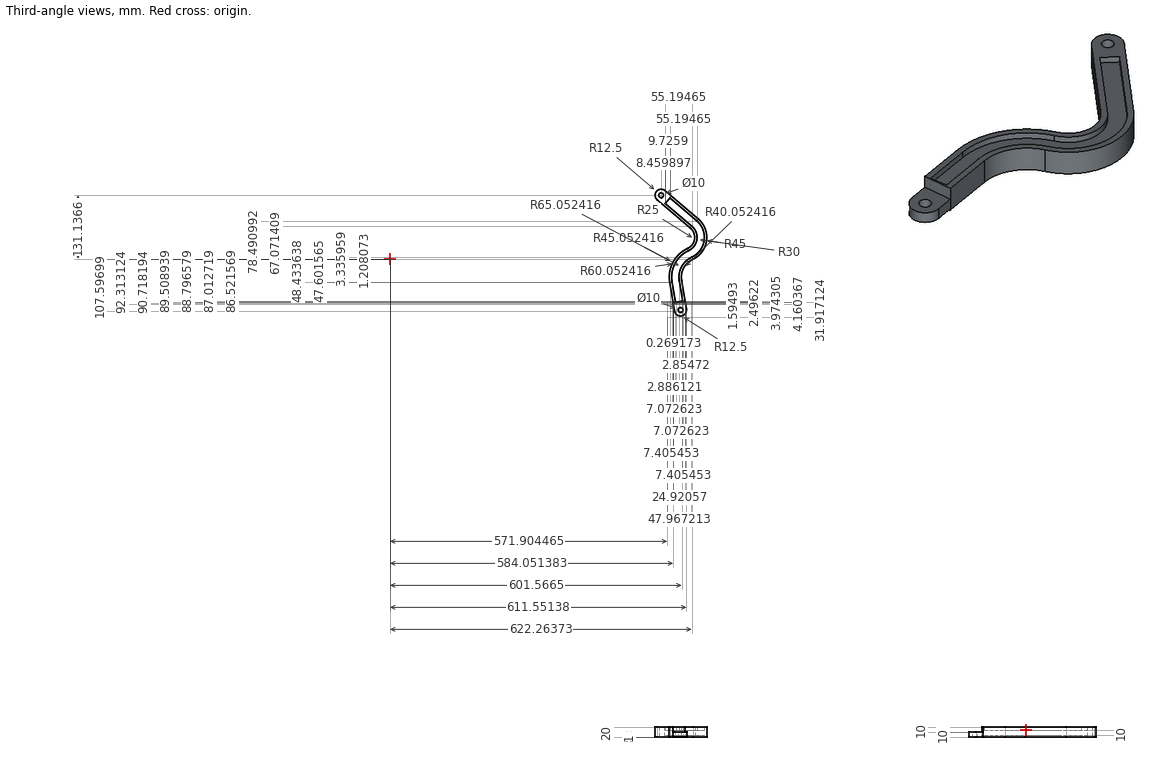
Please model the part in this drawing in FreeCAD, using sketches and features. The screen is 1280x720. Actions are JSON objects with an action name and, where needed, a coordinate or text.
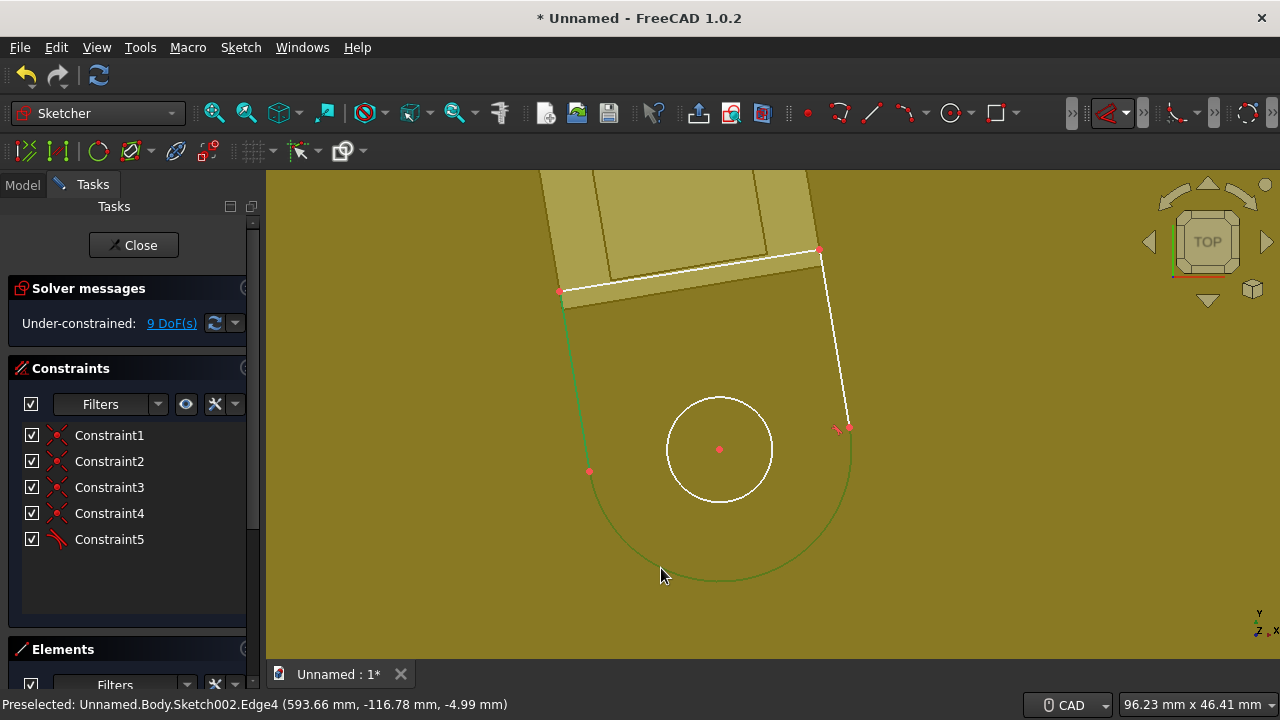
{"action": "key", "text": "t"}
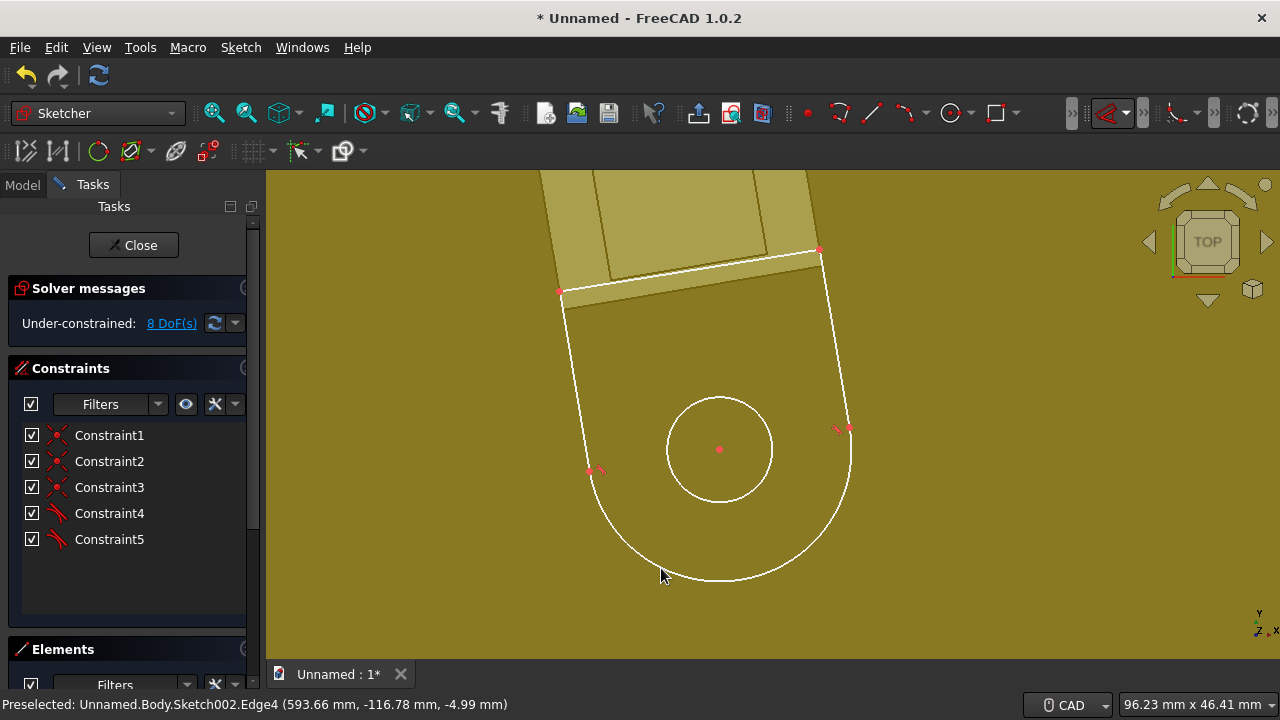
{"action": "left_click", "coordinate": [661, 568]}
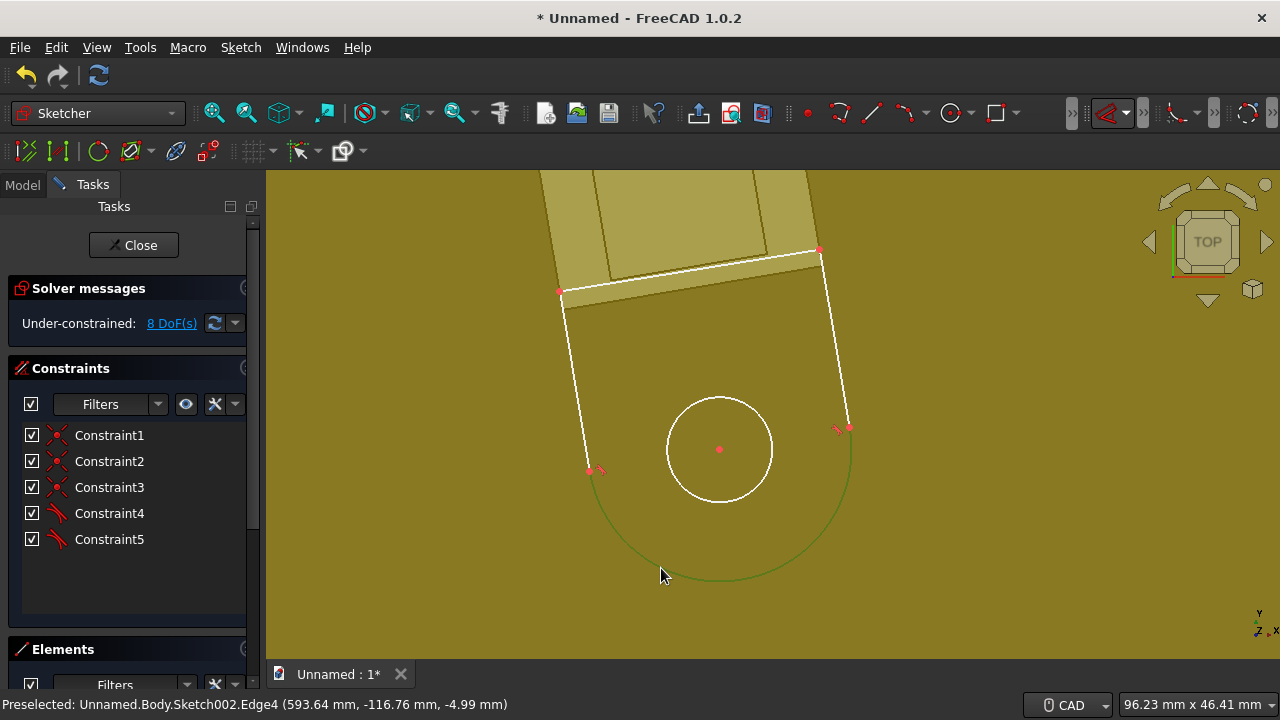
{"action": "left_click", "coordinate": [1128, 114]}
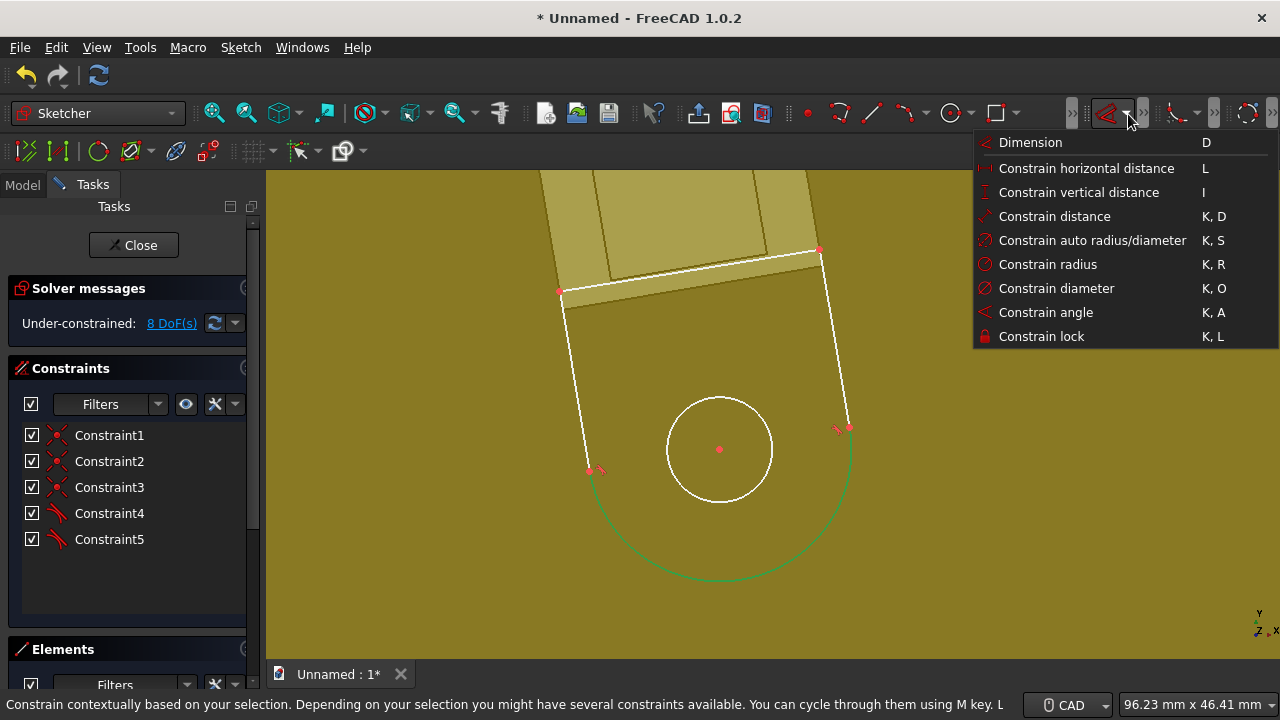
{"action": "left_click", "coordinate": [1126, 264]}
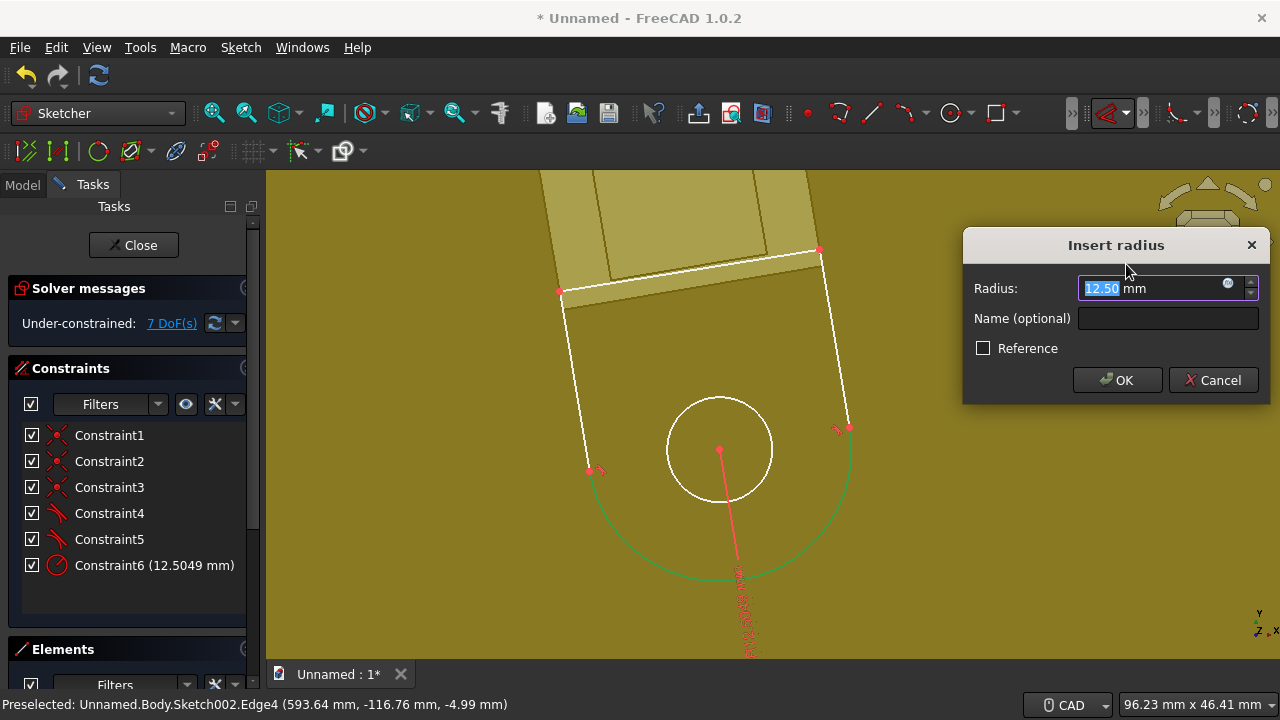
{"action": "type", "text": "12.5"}
{"action": "key", "text": "Return"}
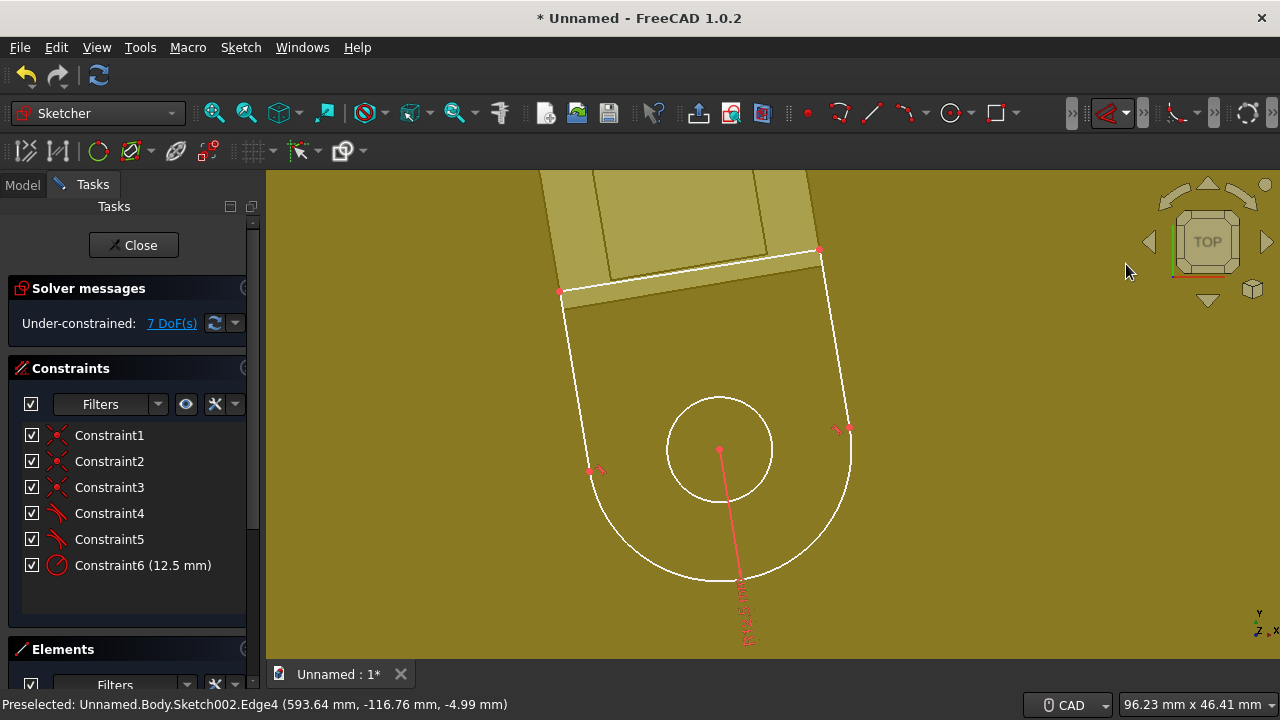
{"action": "left_click", "coordinate": [757, 412]}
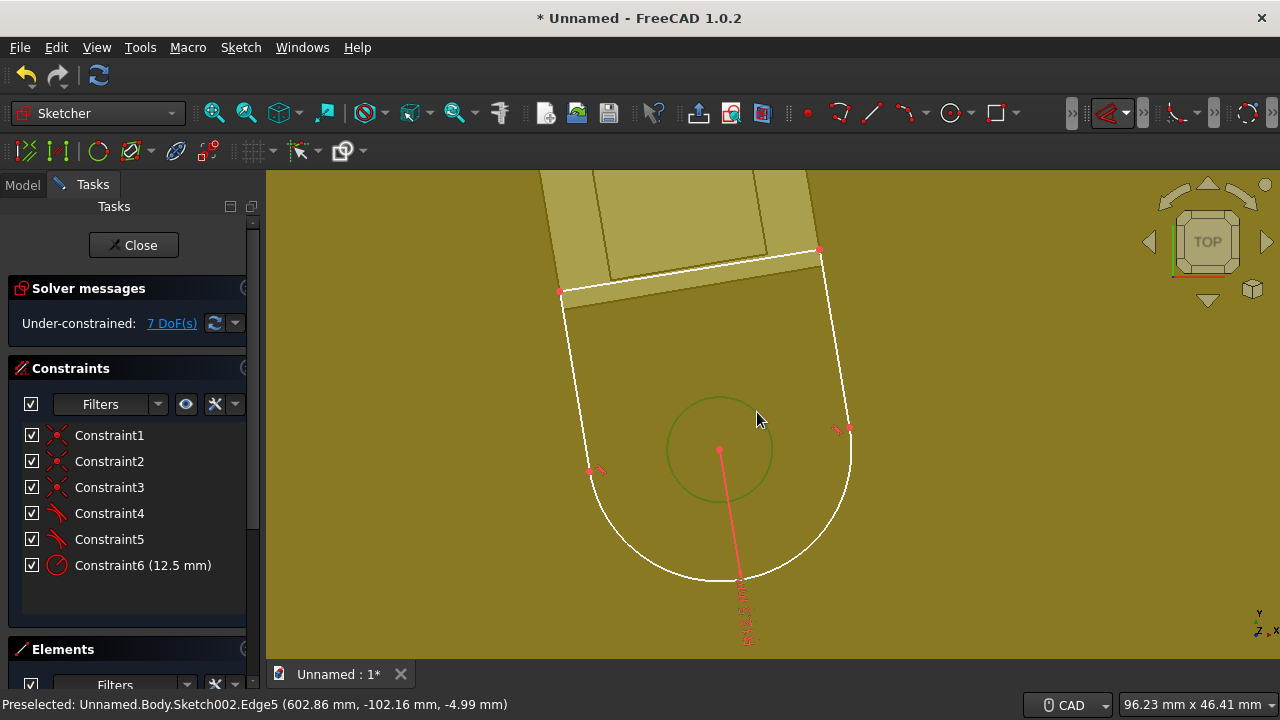
{"action": "left_click", "coordinate": [1128, 114]}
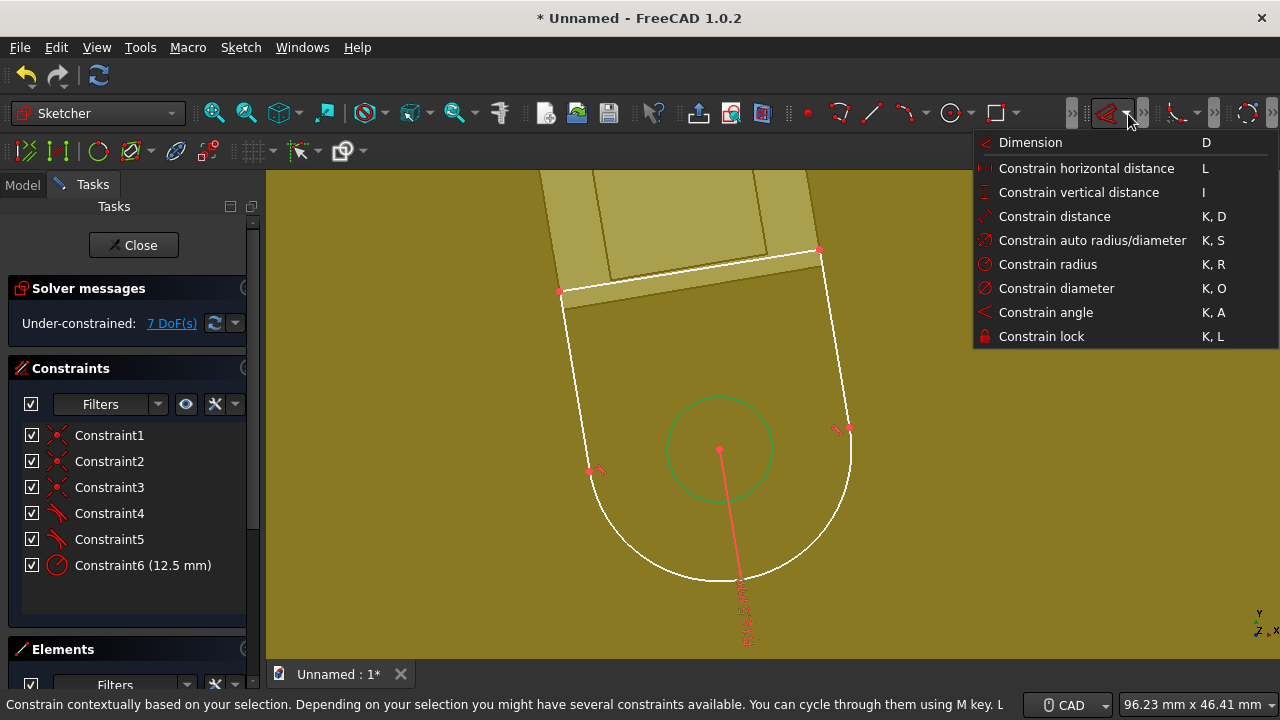
{"action": "left_click", "coordinate": [1126, 288]}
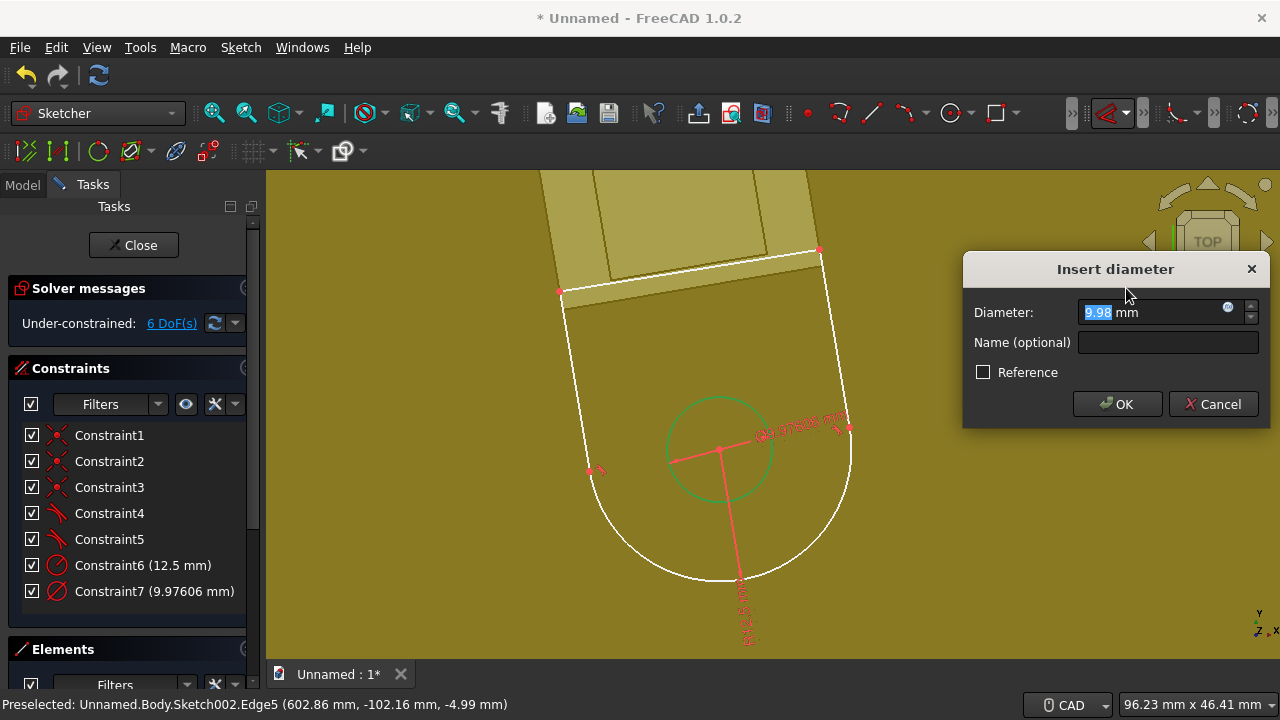
{"action": "type", "text": "10"}
{"action": "key", "text": "Return"}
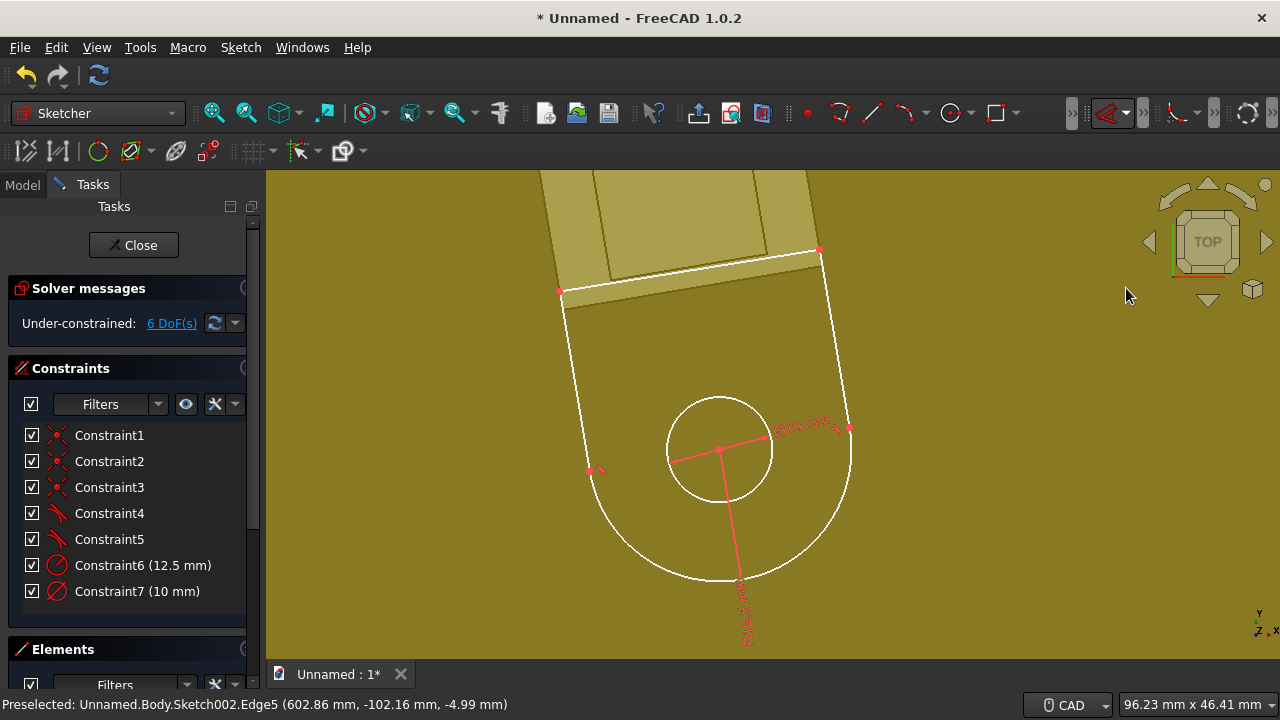
{"action": "scroll", "coordinate": [841, 374], "scroll_direction": "up", "scroll_amount": 2}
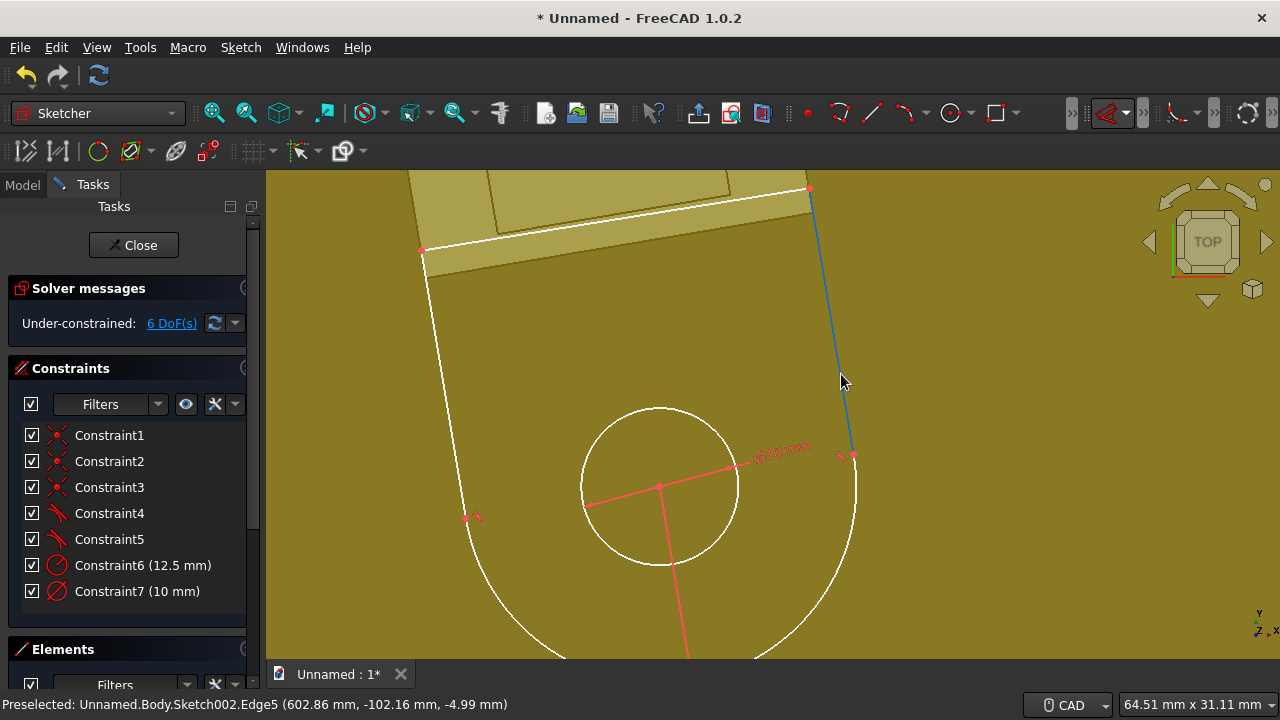
{"action": "left_click", "coordinate": [840, 374]}